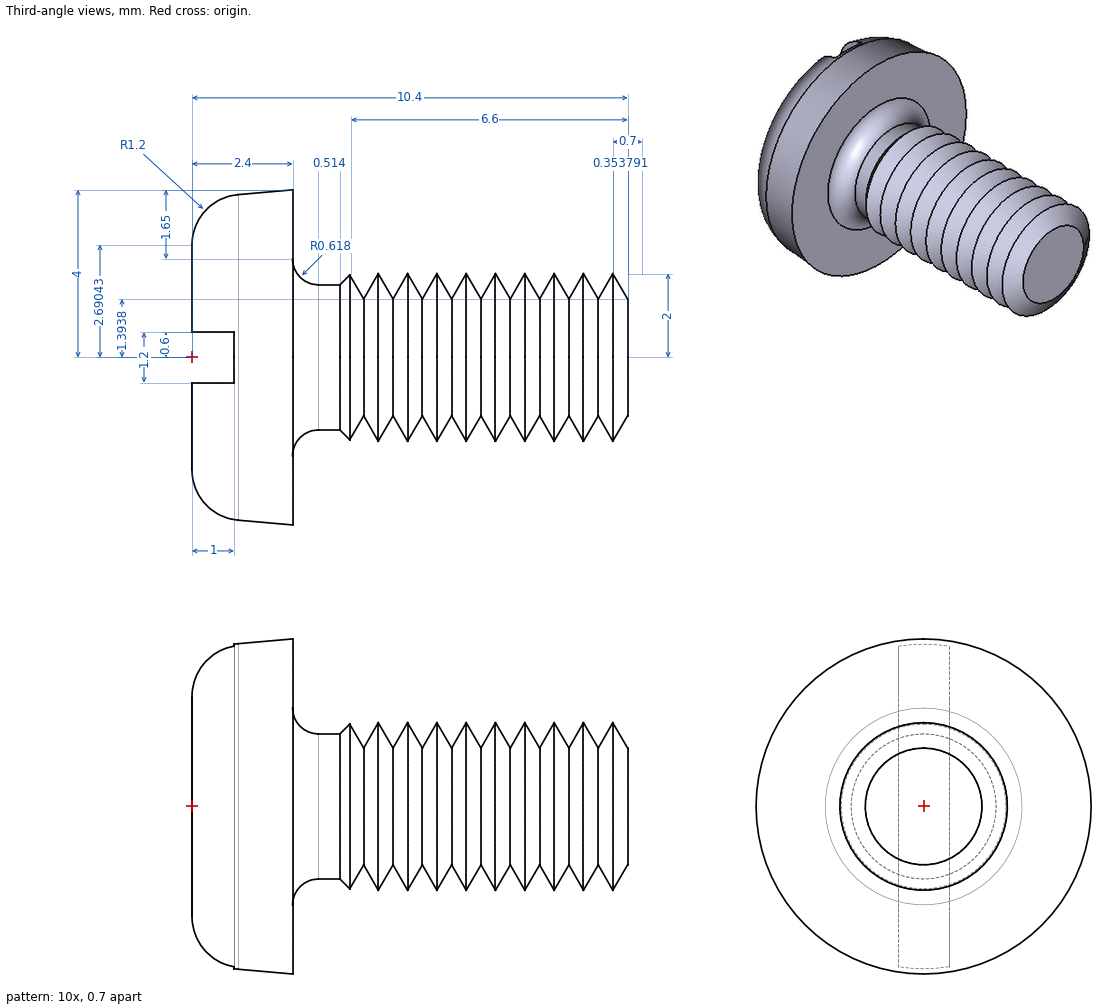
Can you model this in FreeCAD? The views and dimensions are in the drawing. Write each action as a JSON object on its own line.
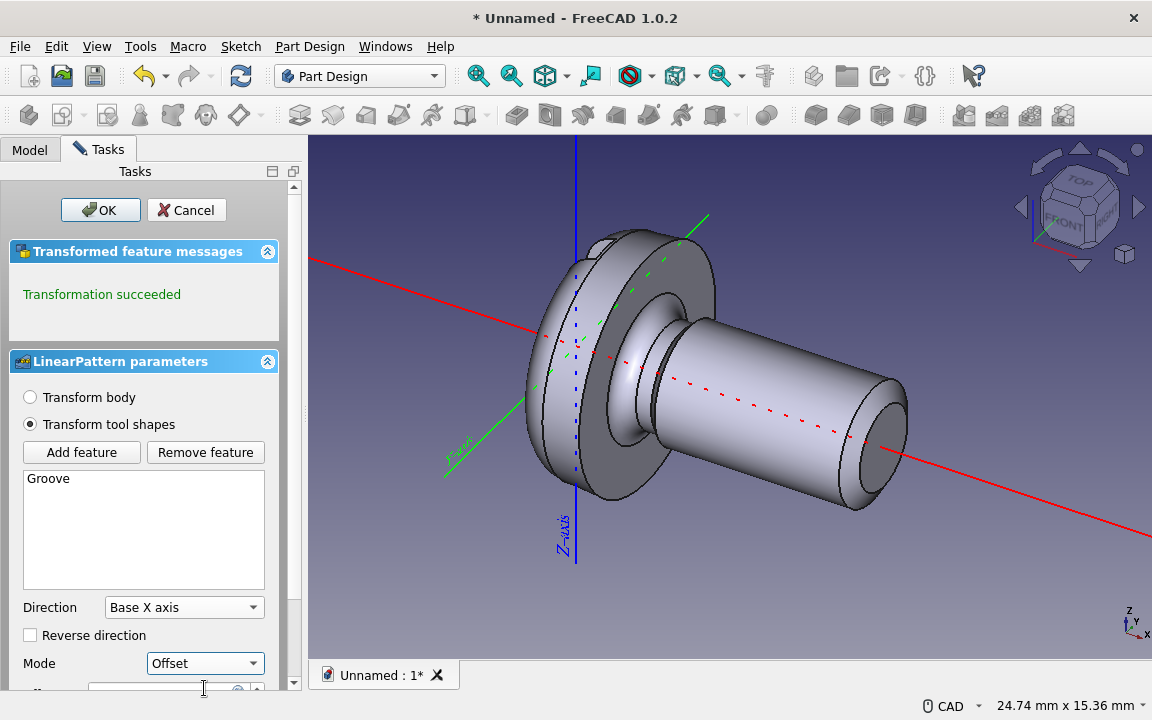
{"action": "scroll", "coordinate": [294, 436], "scroll_direction": "down", "scroll_amount": 2}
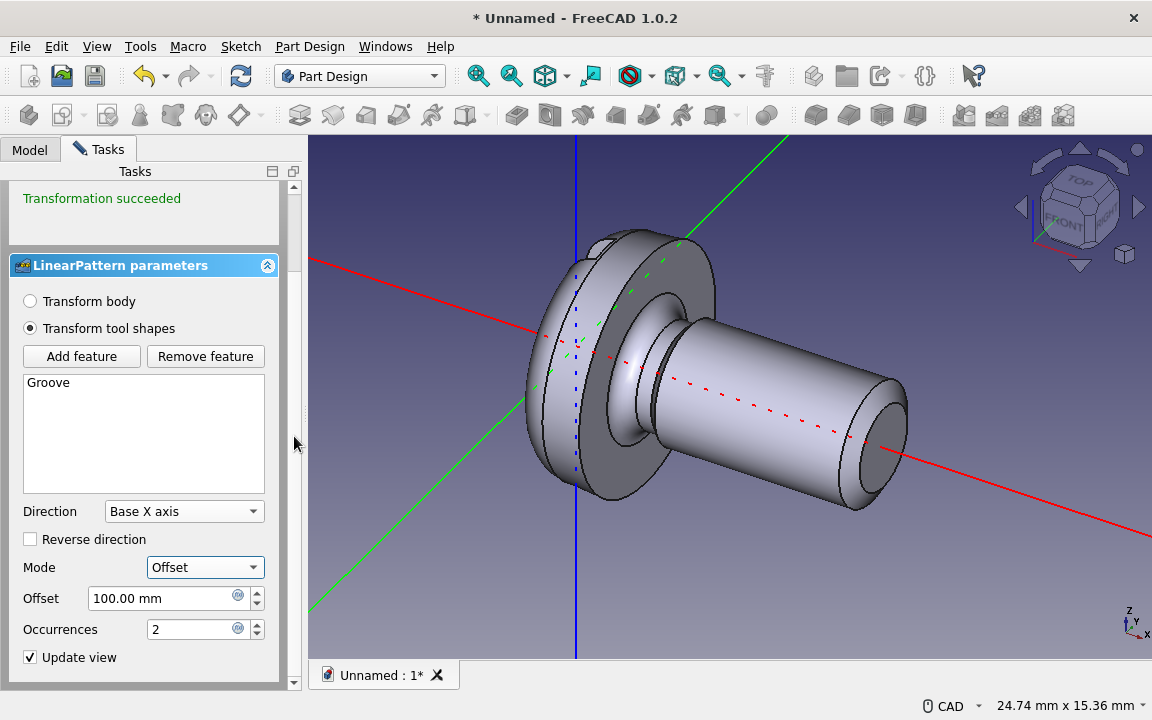
{"action": "triple_click", "coordinate": [170, 598]}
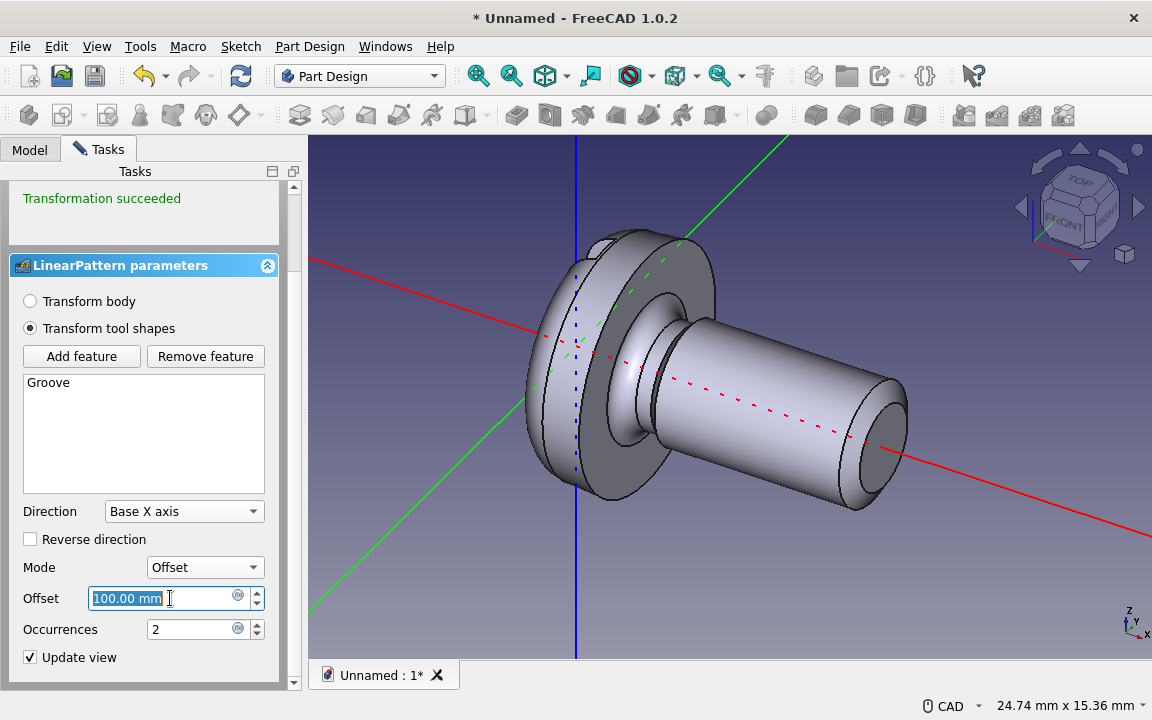
{"action": "type", "text": "0.7"}
{"action": "key", "text": "Tab"}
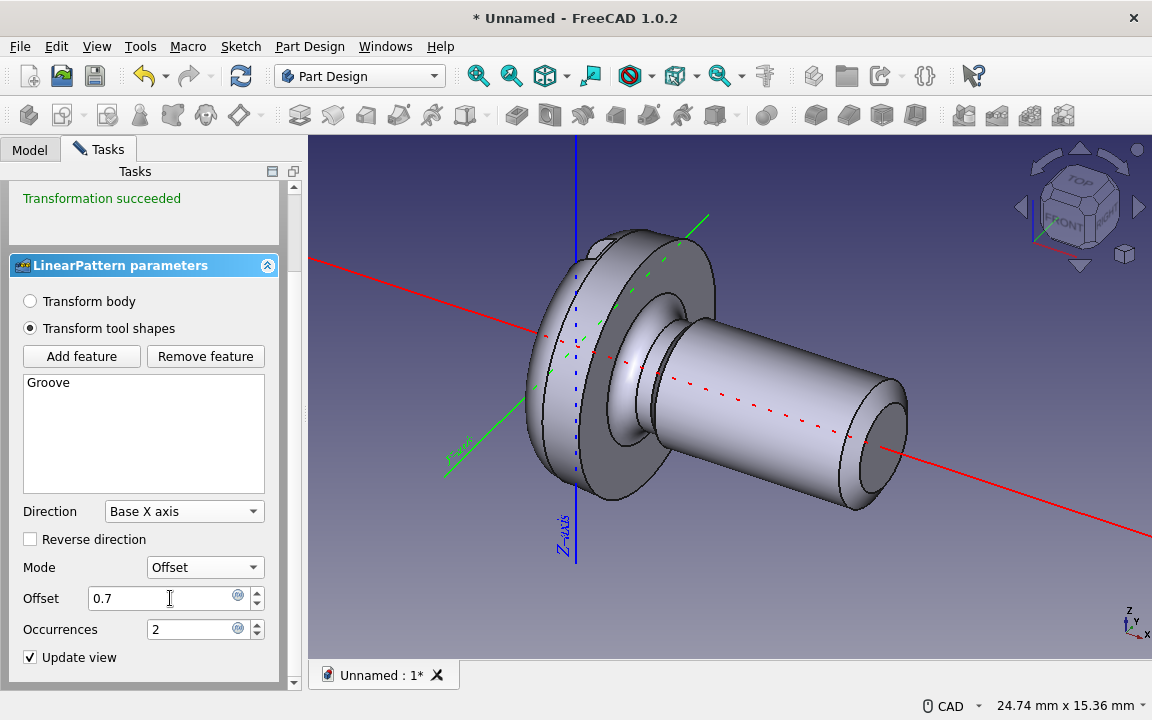
{"action": "triple_click", "coordinate": [199, 630]}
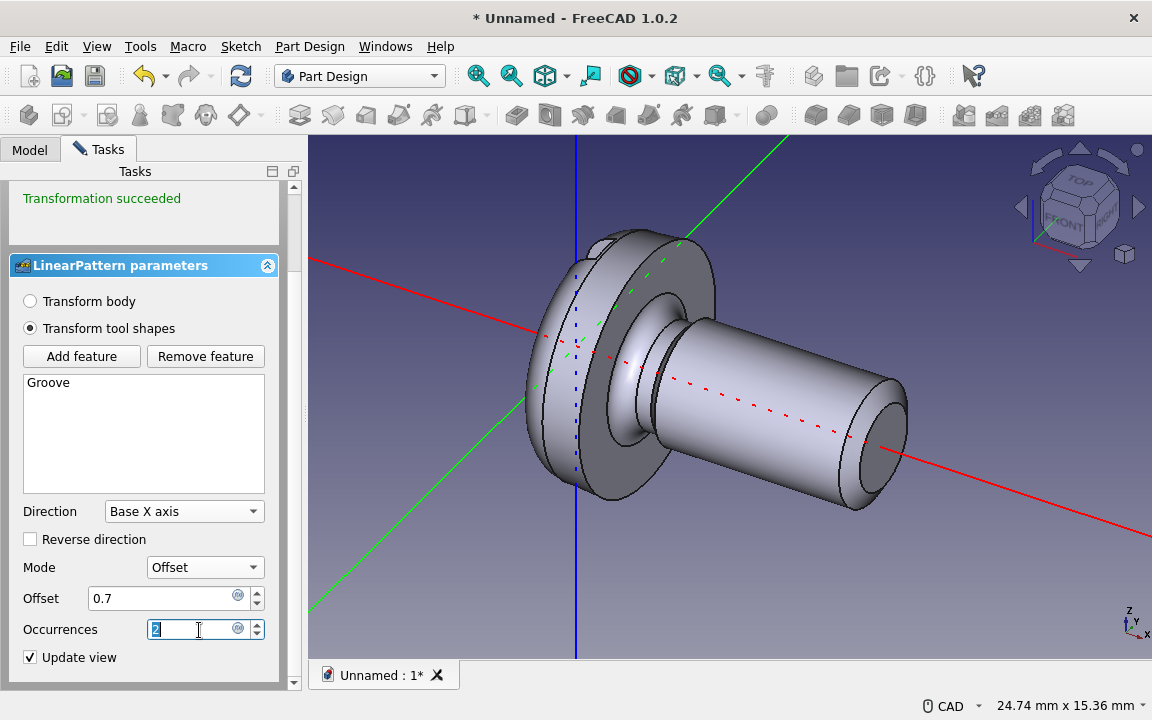
{"action": "type", "text": "10"}
{"action": "key", "text": "Tab"}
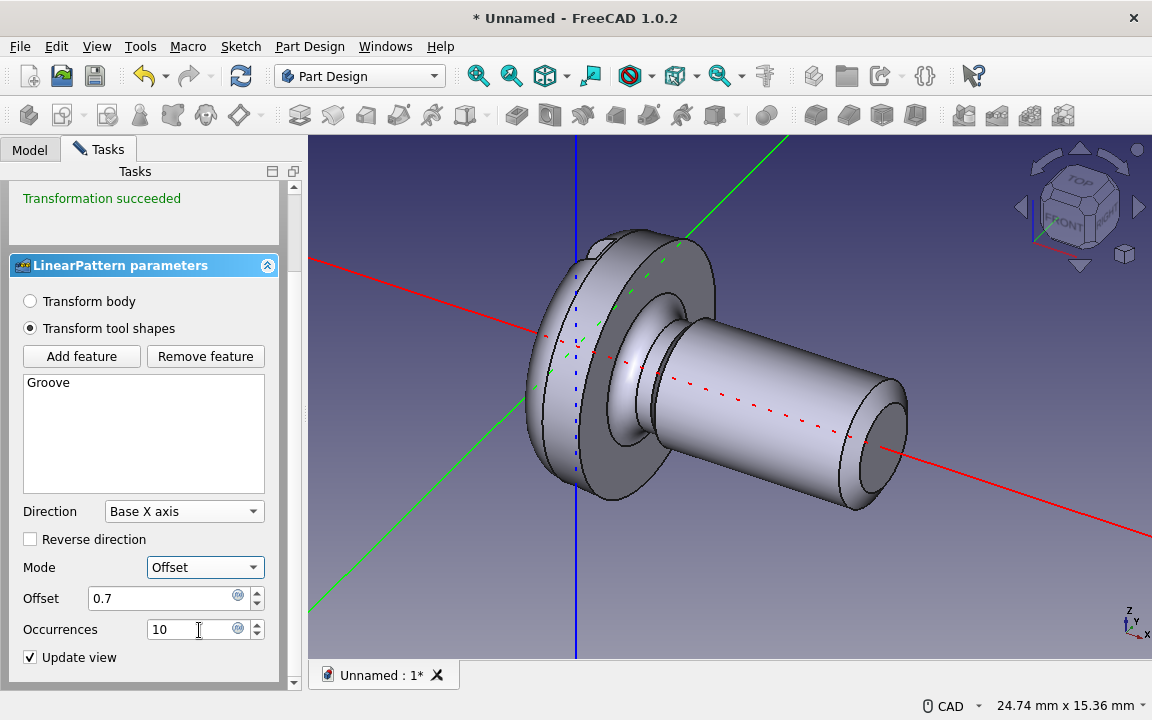
{"action": "left_click", "coordinate": [31, 539]}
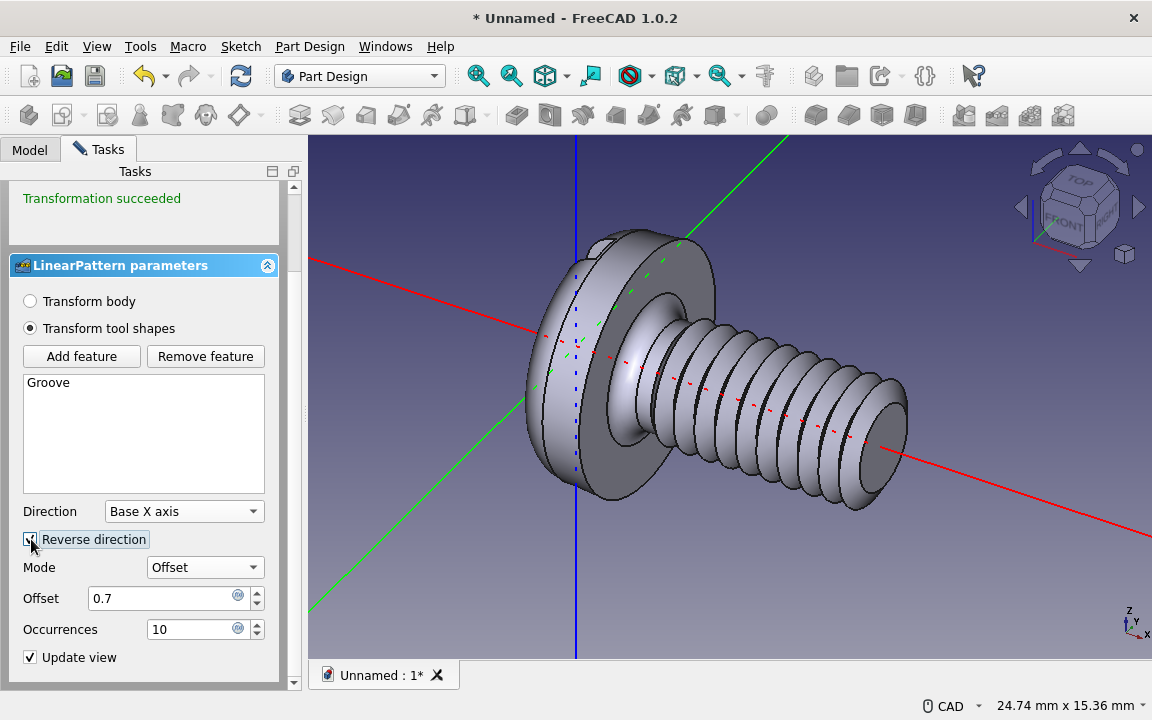
{"action": "scroll", "coordinate": [294, 436], "scroll_direction": "up", "scroll_amount": 3}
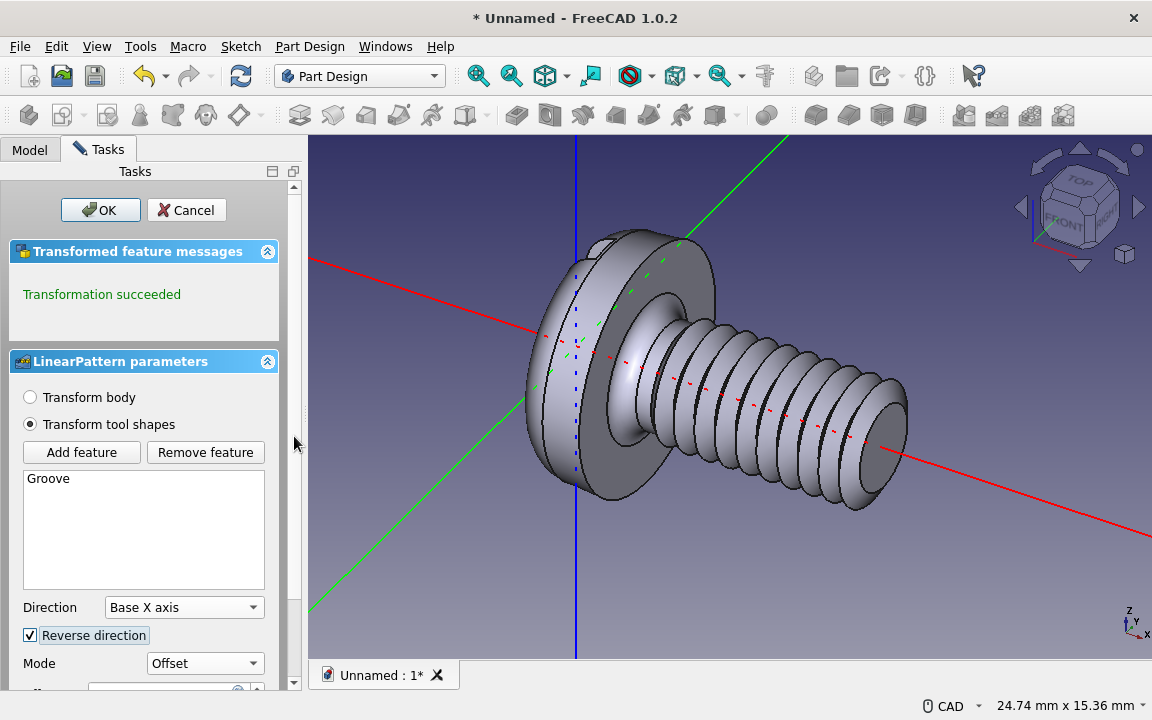
{"action": "left_click", "coordinate": [101, 210]}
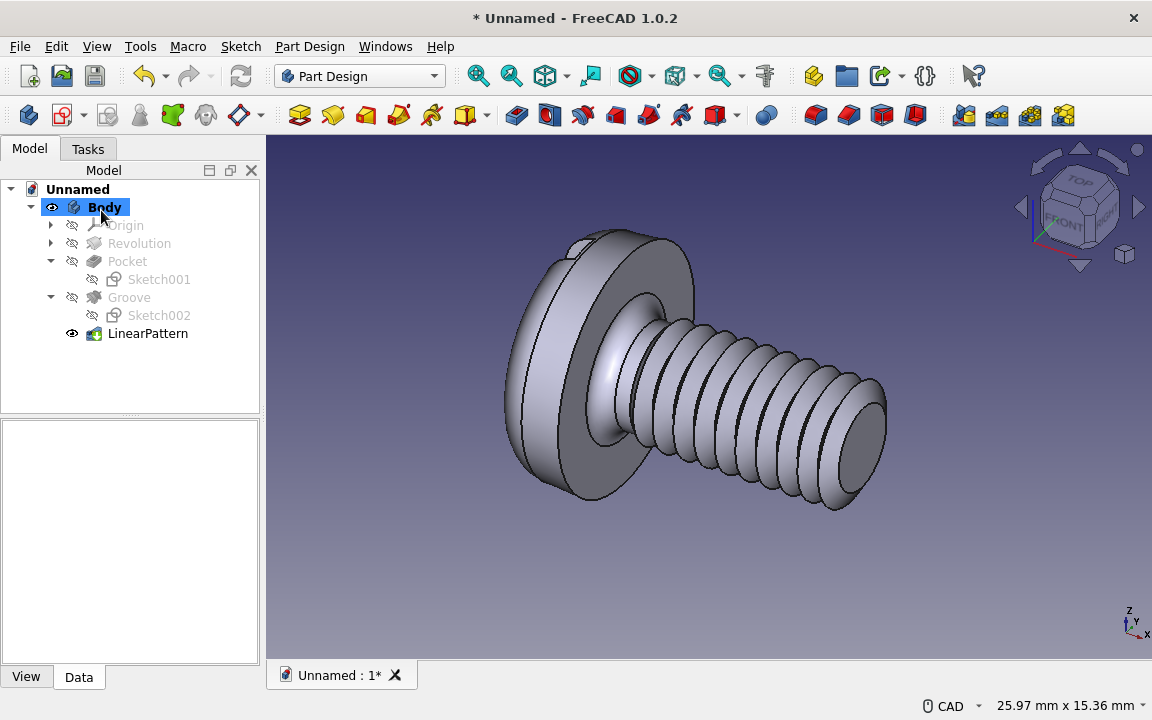
{"action": "key", "text": "0"}